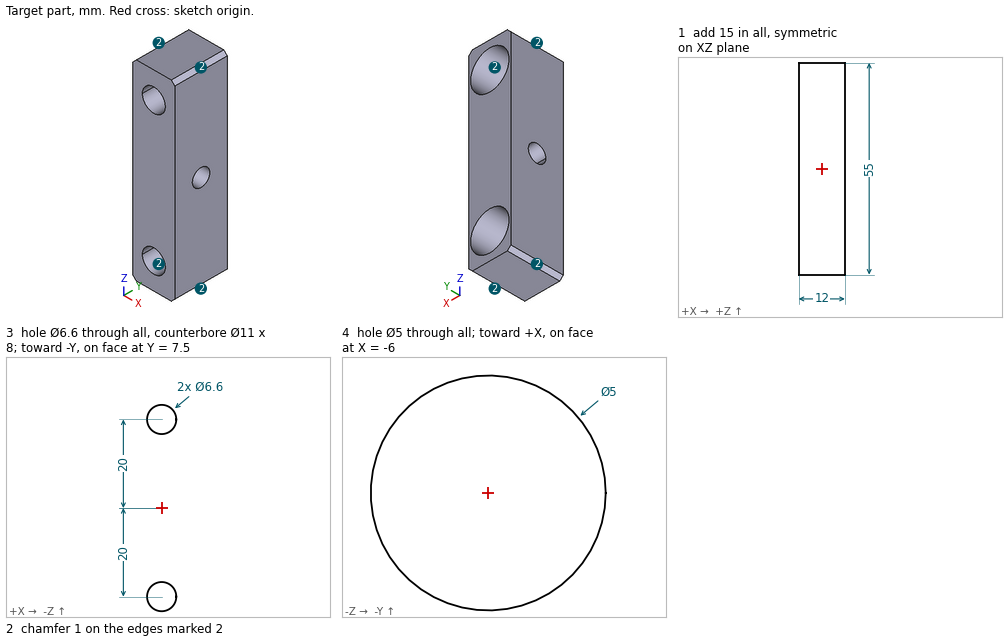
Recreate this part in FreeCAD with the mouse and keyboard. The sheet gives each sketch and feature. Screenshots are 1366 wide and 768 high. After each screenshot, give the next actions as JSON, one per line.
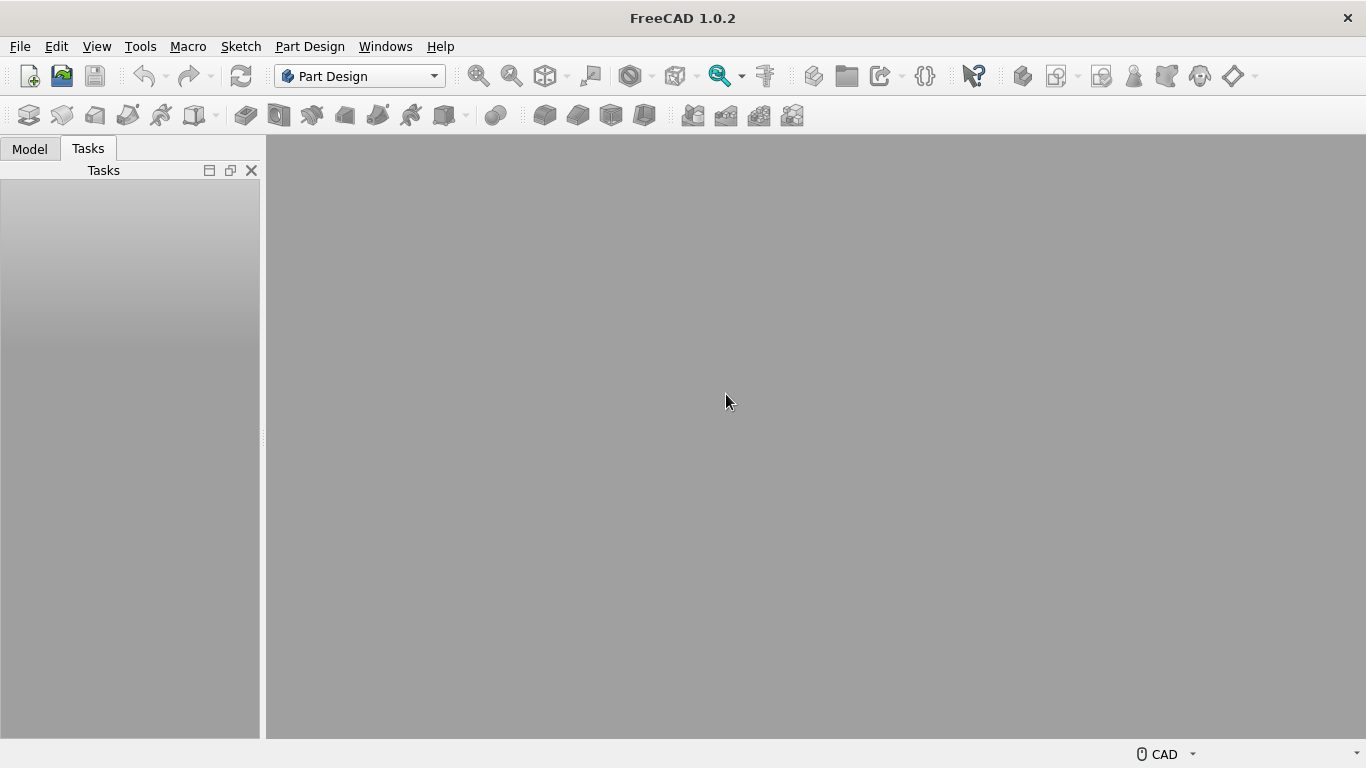
{"action": "left_click", "coordinate": [29, 76]}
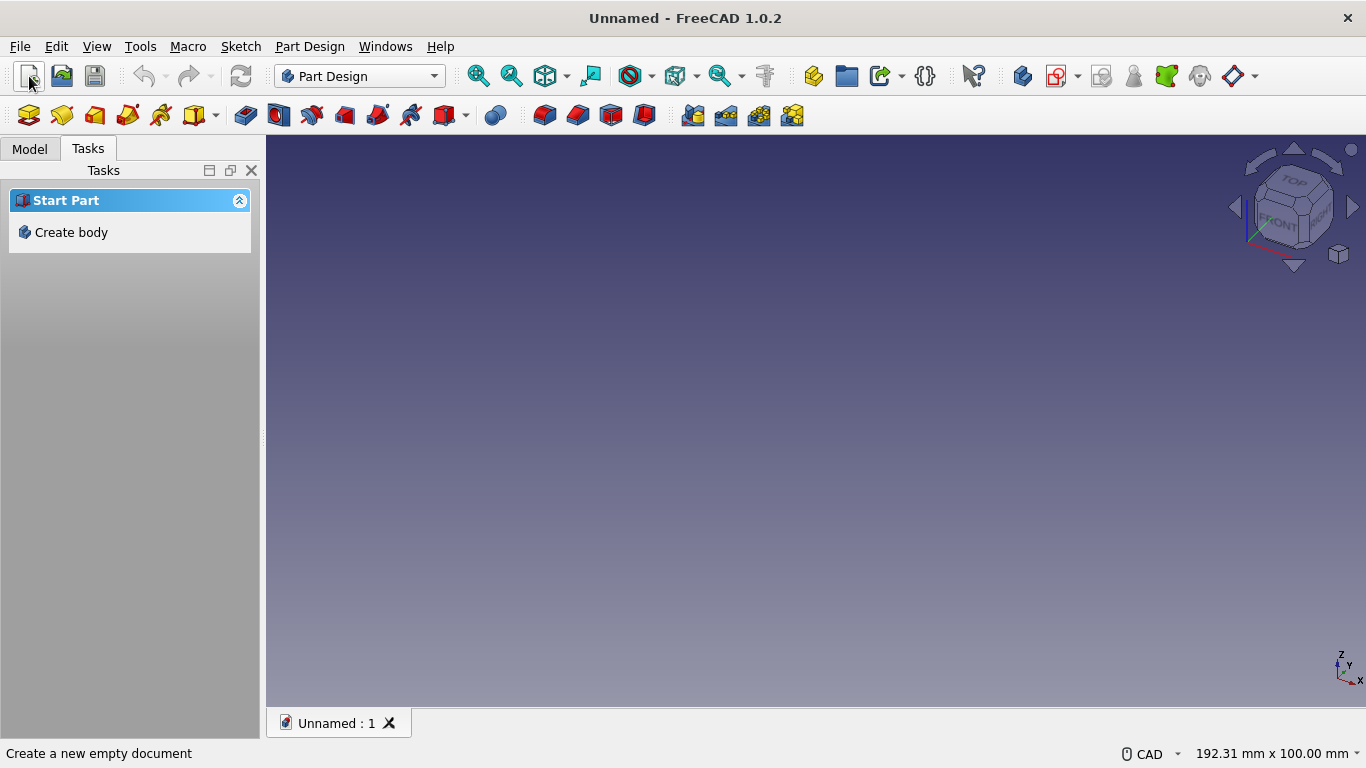
{"action": "left_click", "coordinate": [1056, 76]}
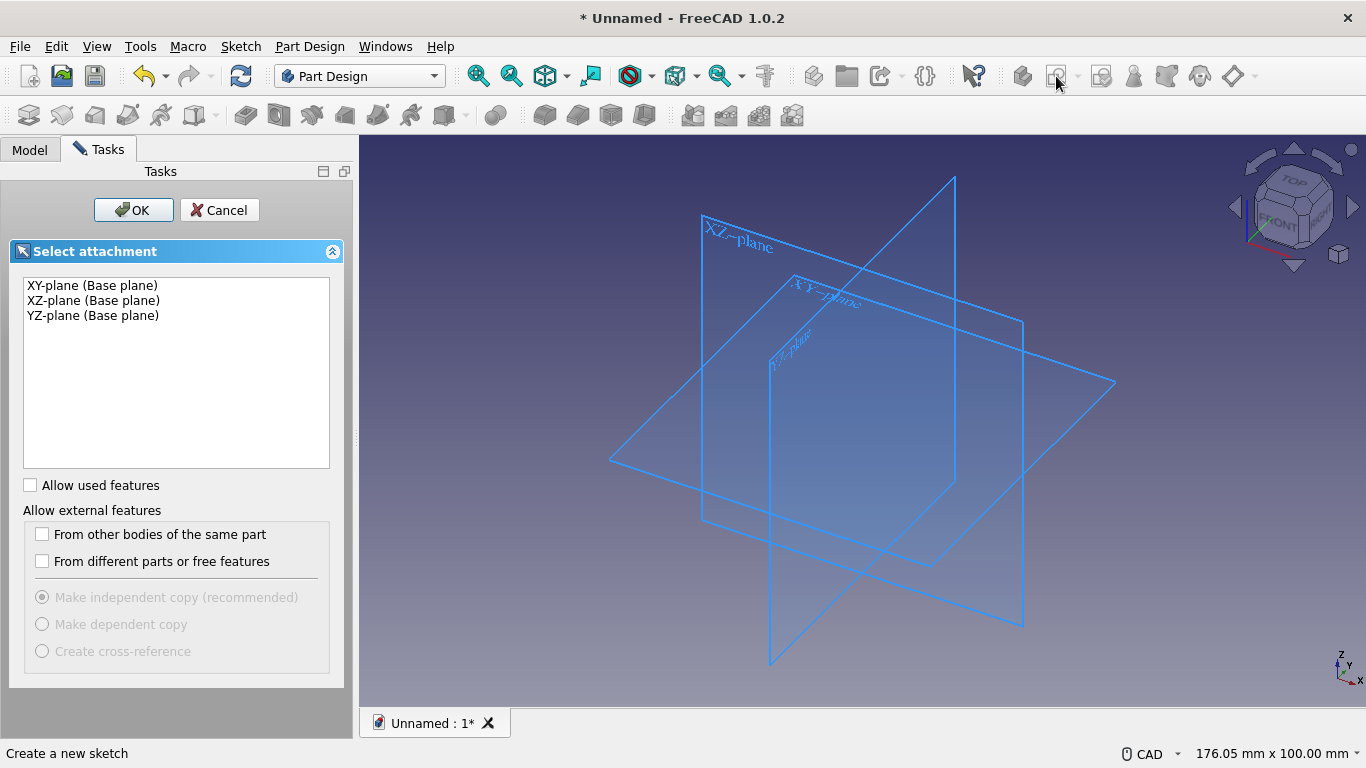
{"action": "left_click", "coordinate": [84, 300]}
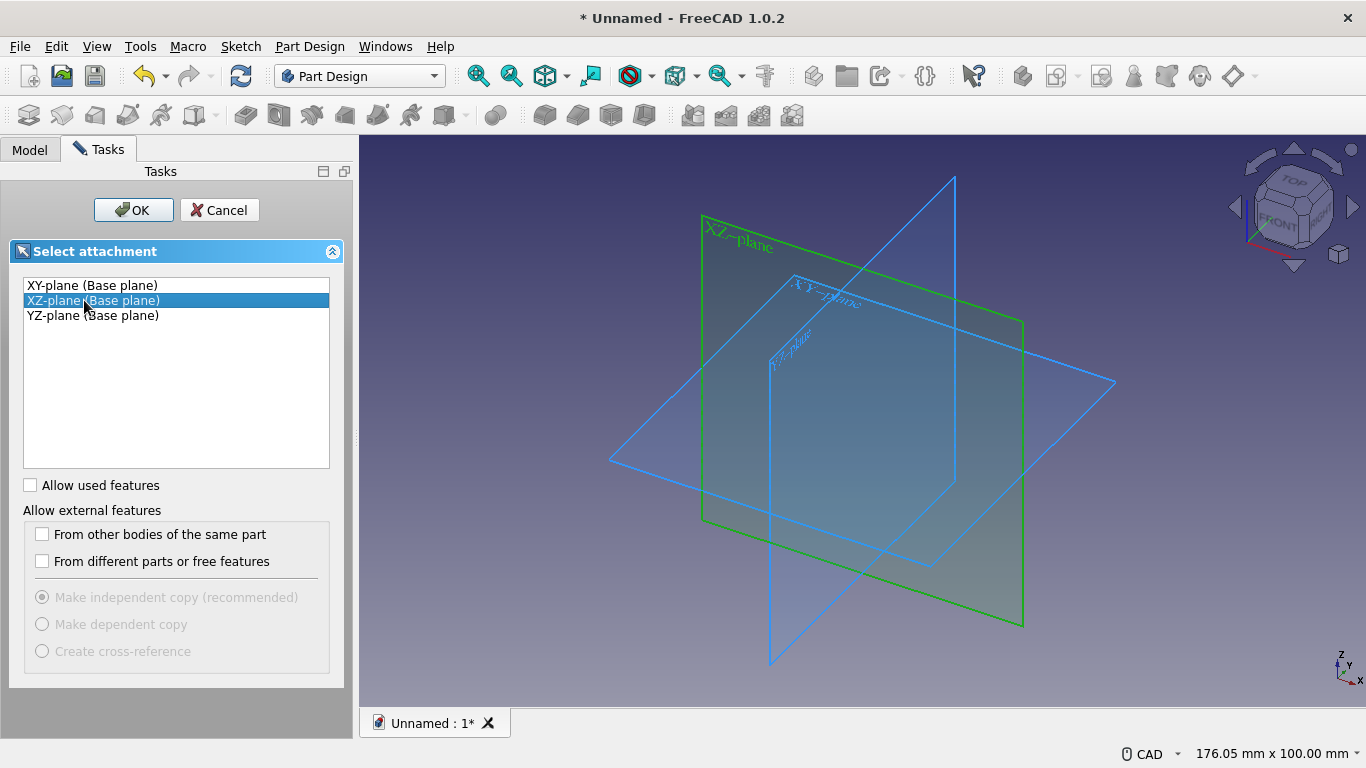
{"action": "left_click", "coordinate": [134, 210]}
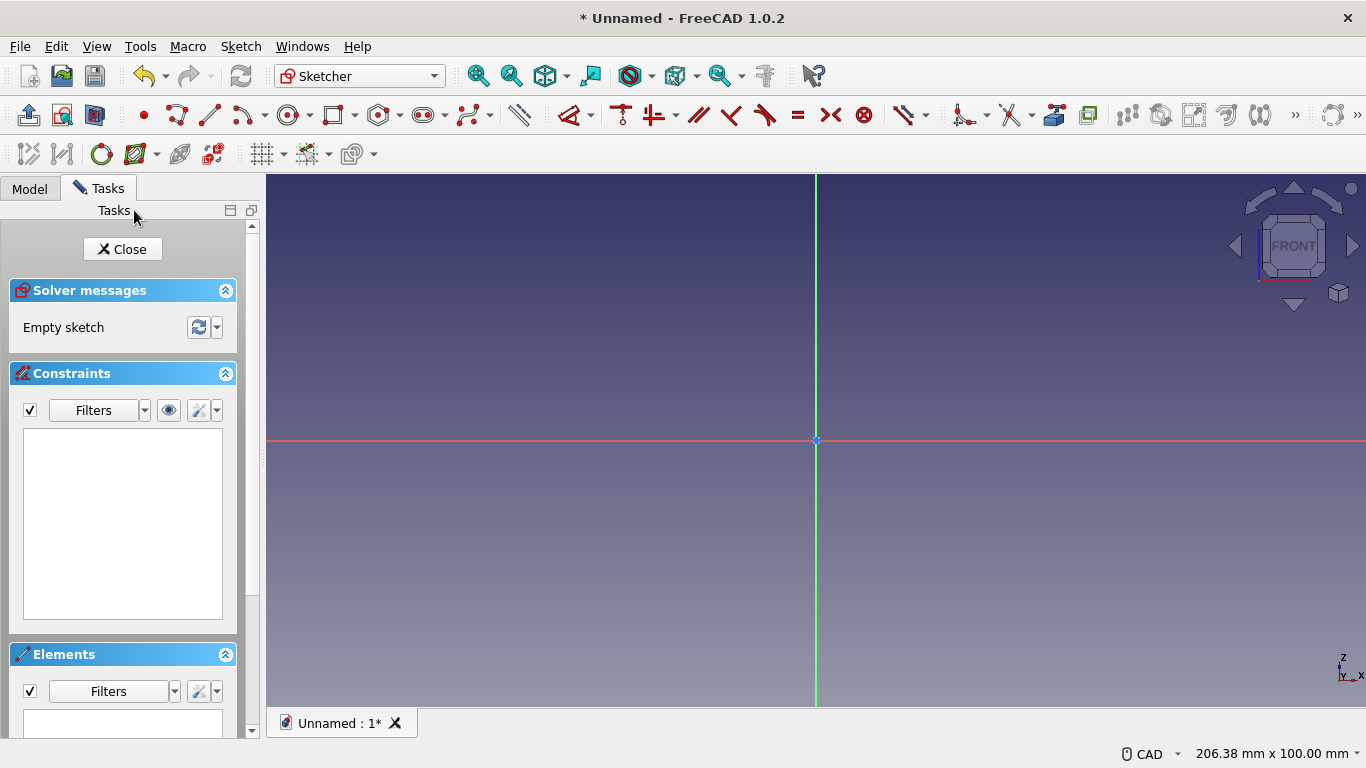
{"action": "left_click", "coordinate": [354, 116]}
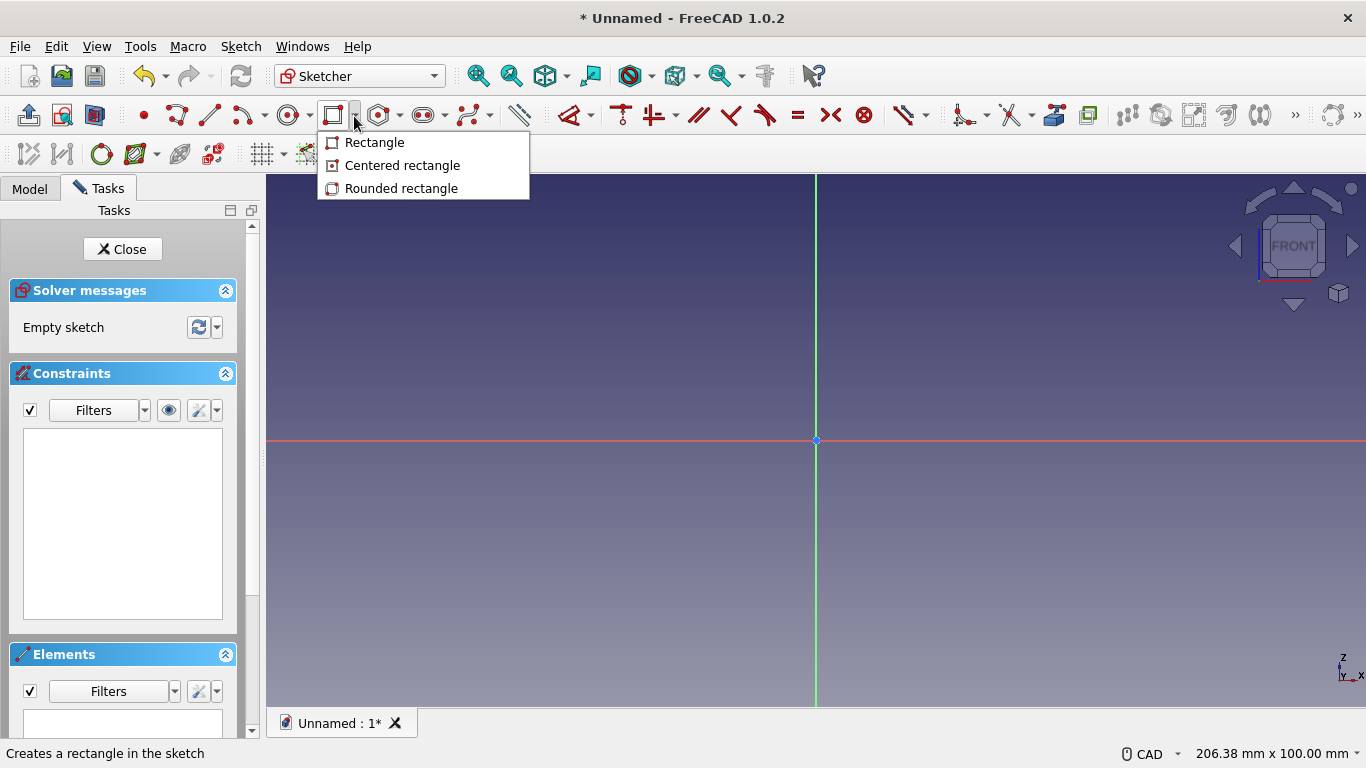
{"action": "left_click", "coordinate": [424, 166]}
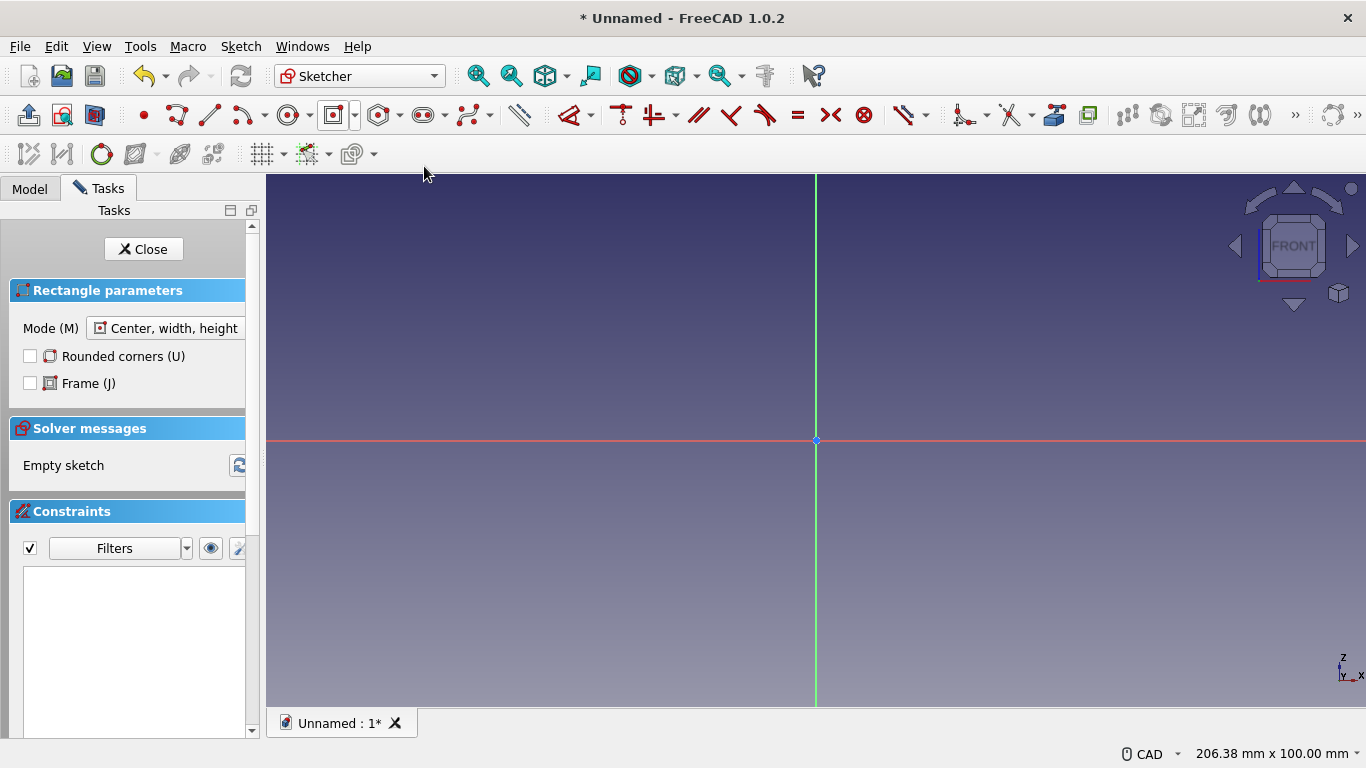
{"action": "left_click", "coordinate": [816, 440]}
{"action": "mouse_move", "coordinate": [848, 294]}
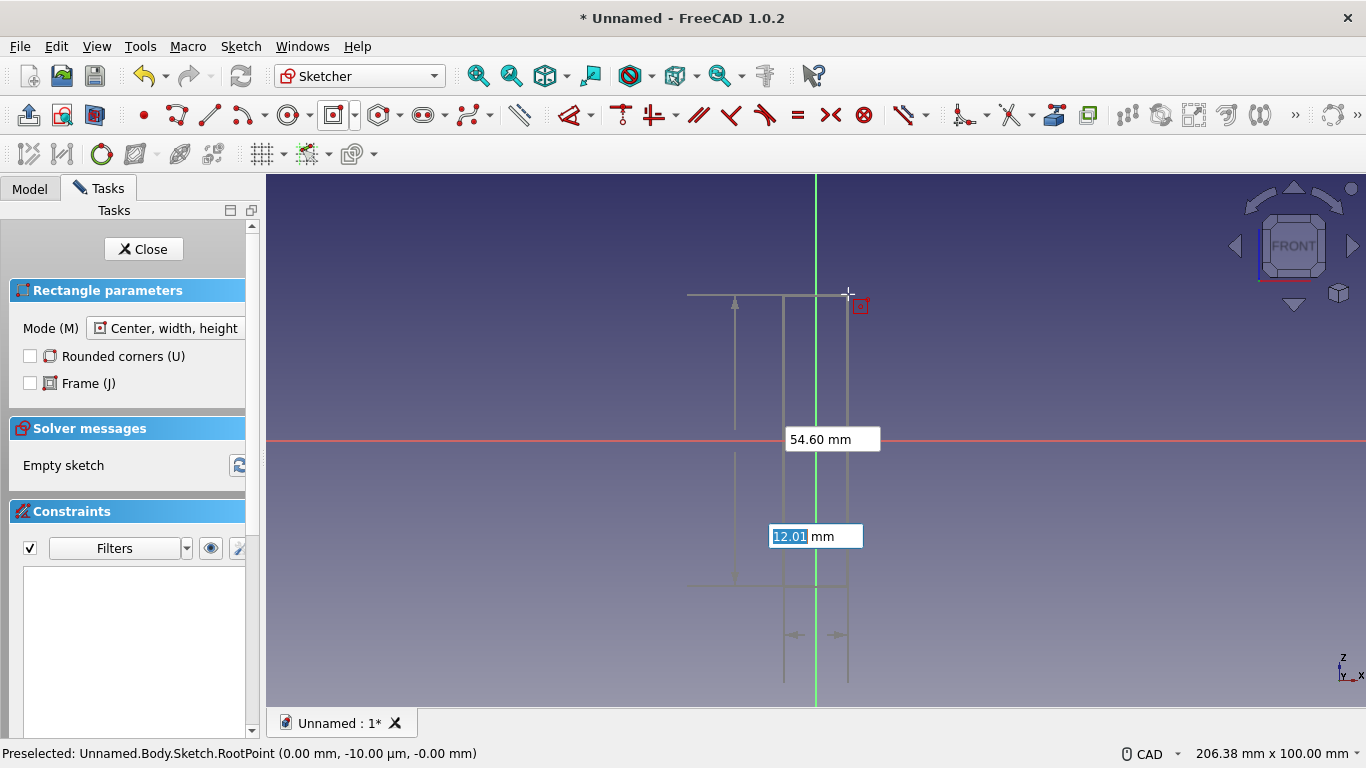
{"action": "type", "text": "12"}
{"action": "key", "text": "Tab"}
{"action": "type", "text": "55"}
{"action": "key", "text": "Return"}
{"action": "key", "text": "Escape"}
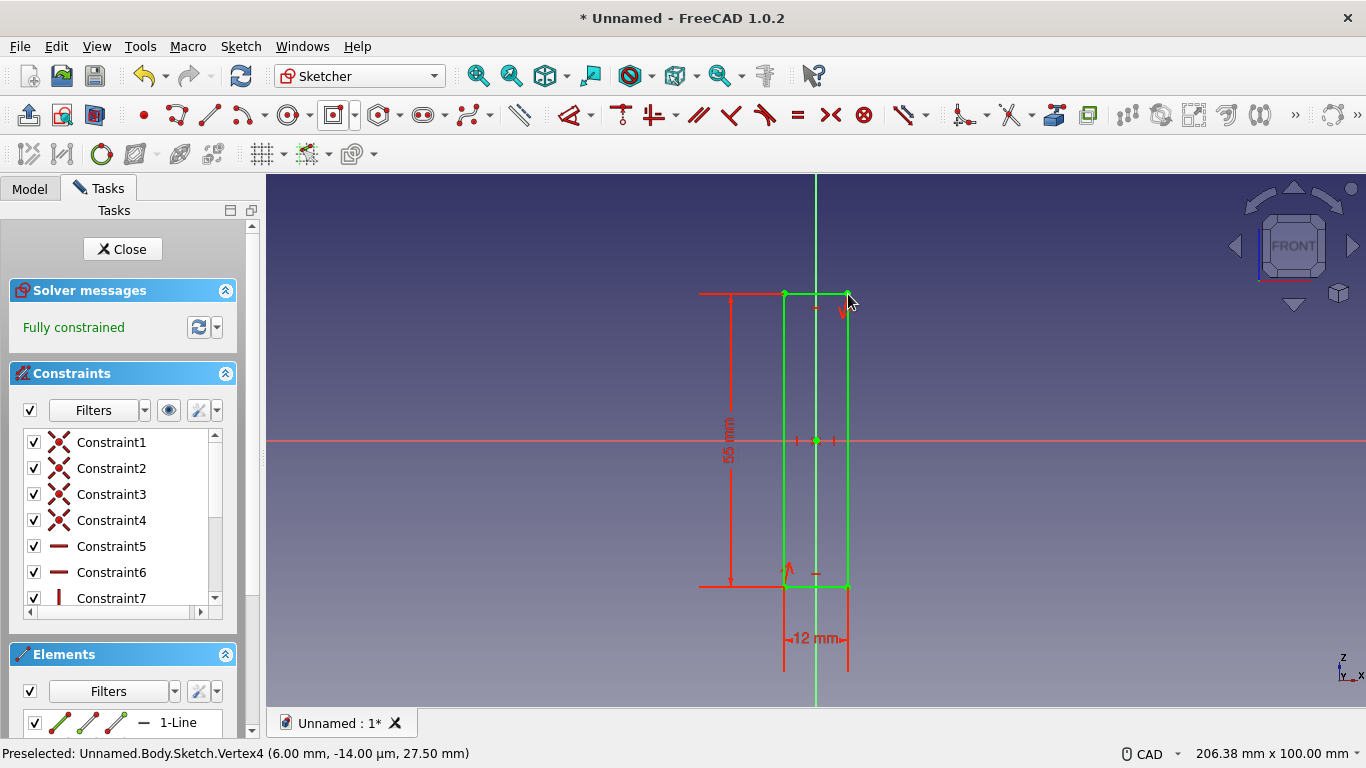
{"action": "left_click", "coordinate": [123, 249]}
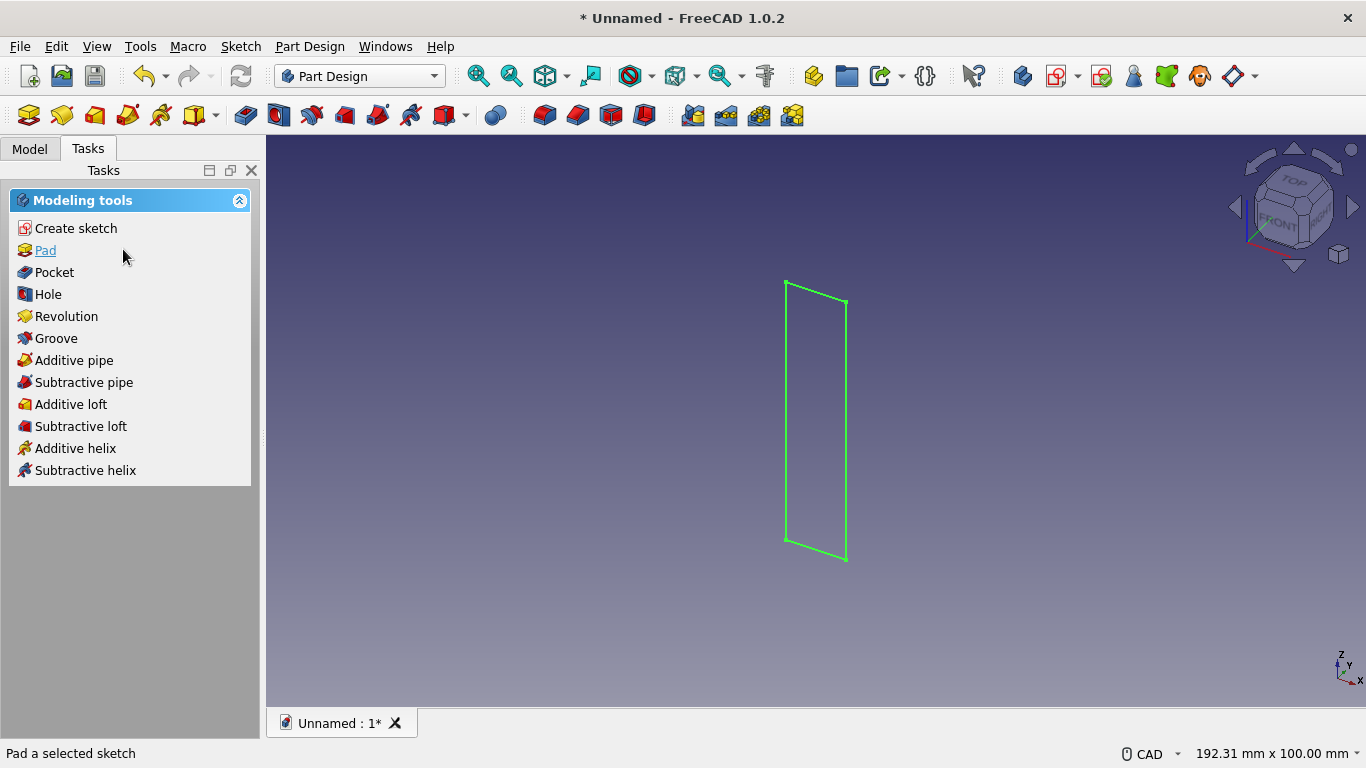
{"action": "left_click", "coordinate": [29, 116]}